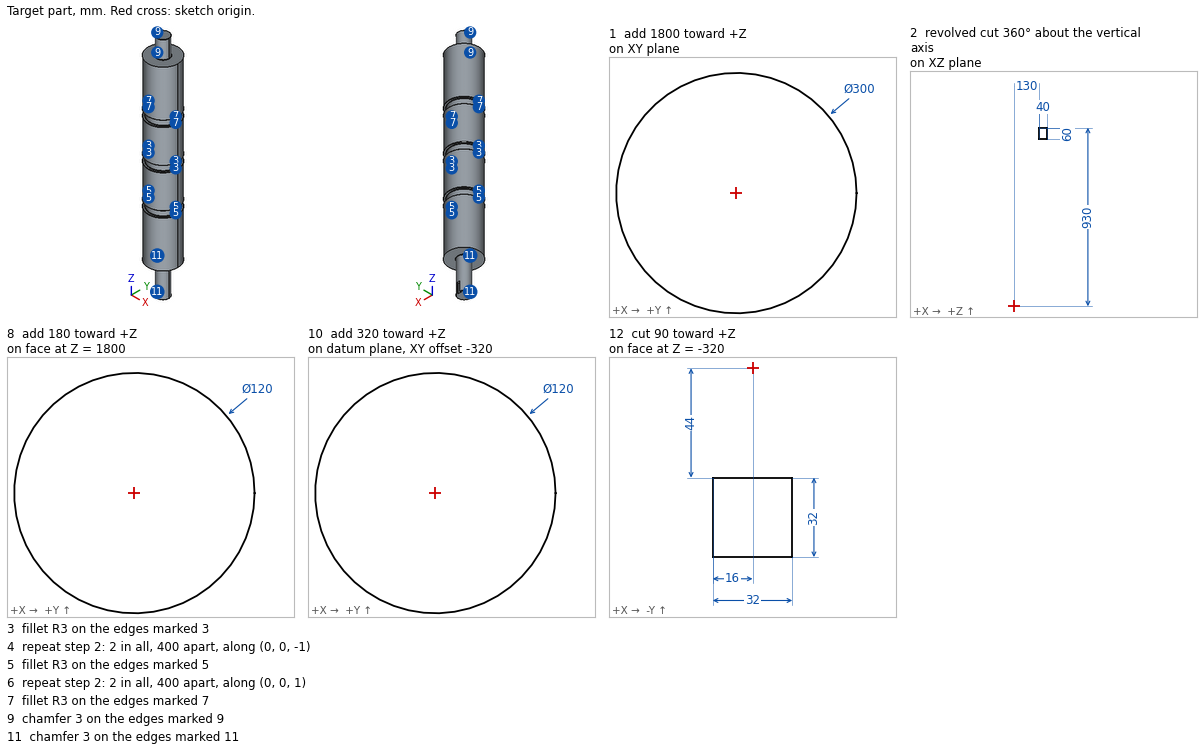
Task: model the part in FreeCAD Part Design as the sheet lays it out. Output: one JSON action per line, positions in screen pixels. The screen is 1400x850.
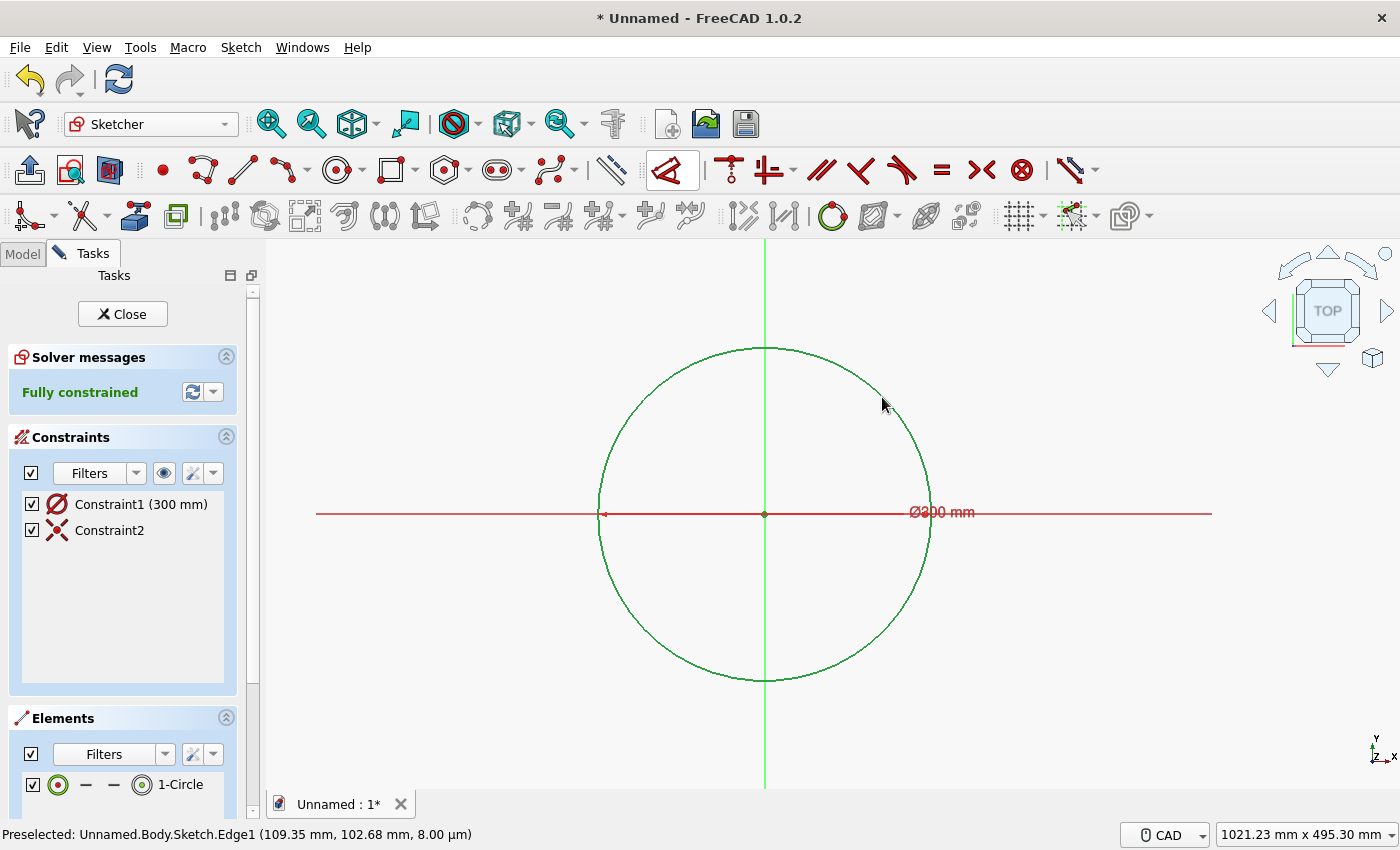
{"action": "left_click", "coordinate": [123, 314]}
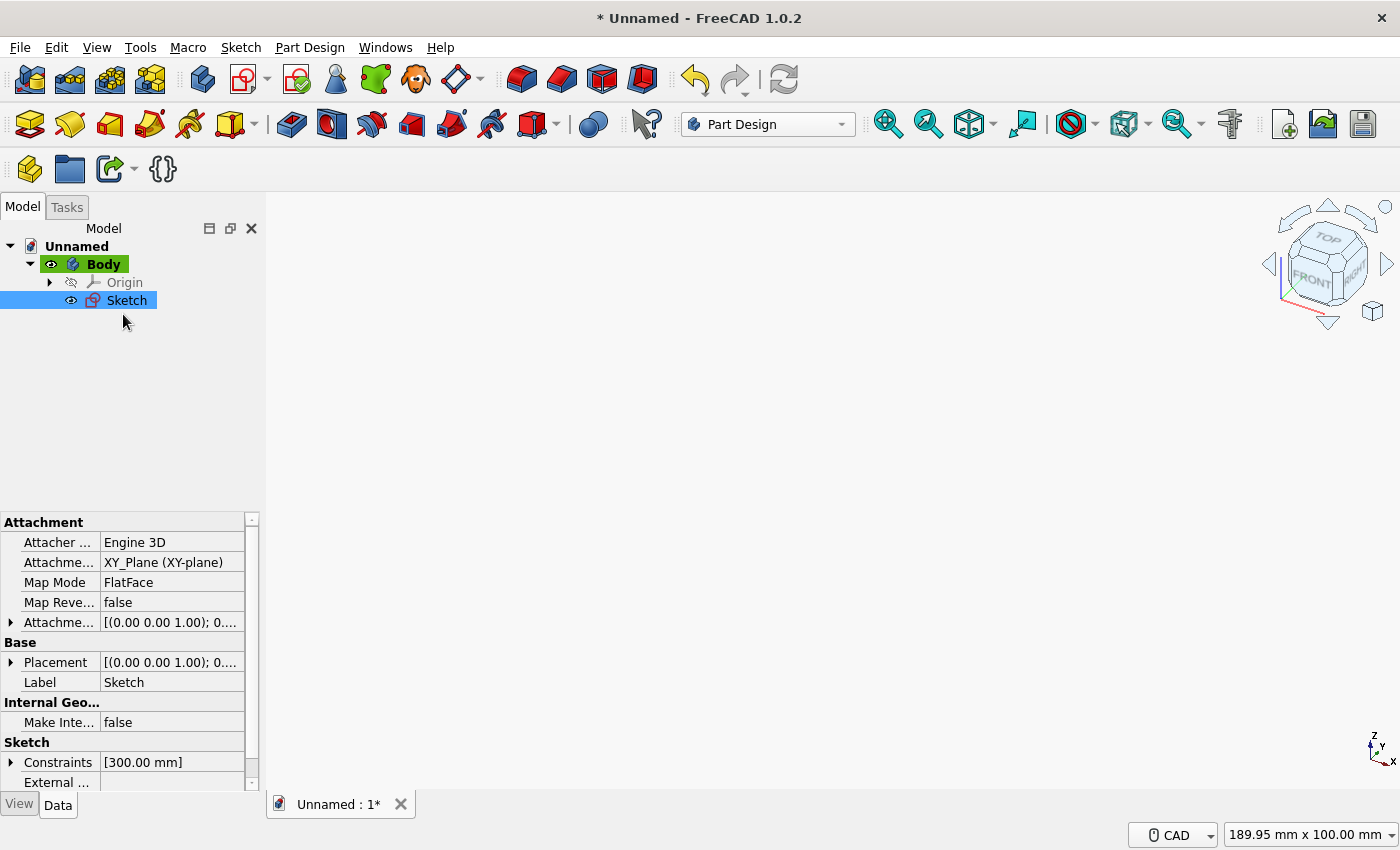
{"action": "left_click", "coordinate": [30, 124]}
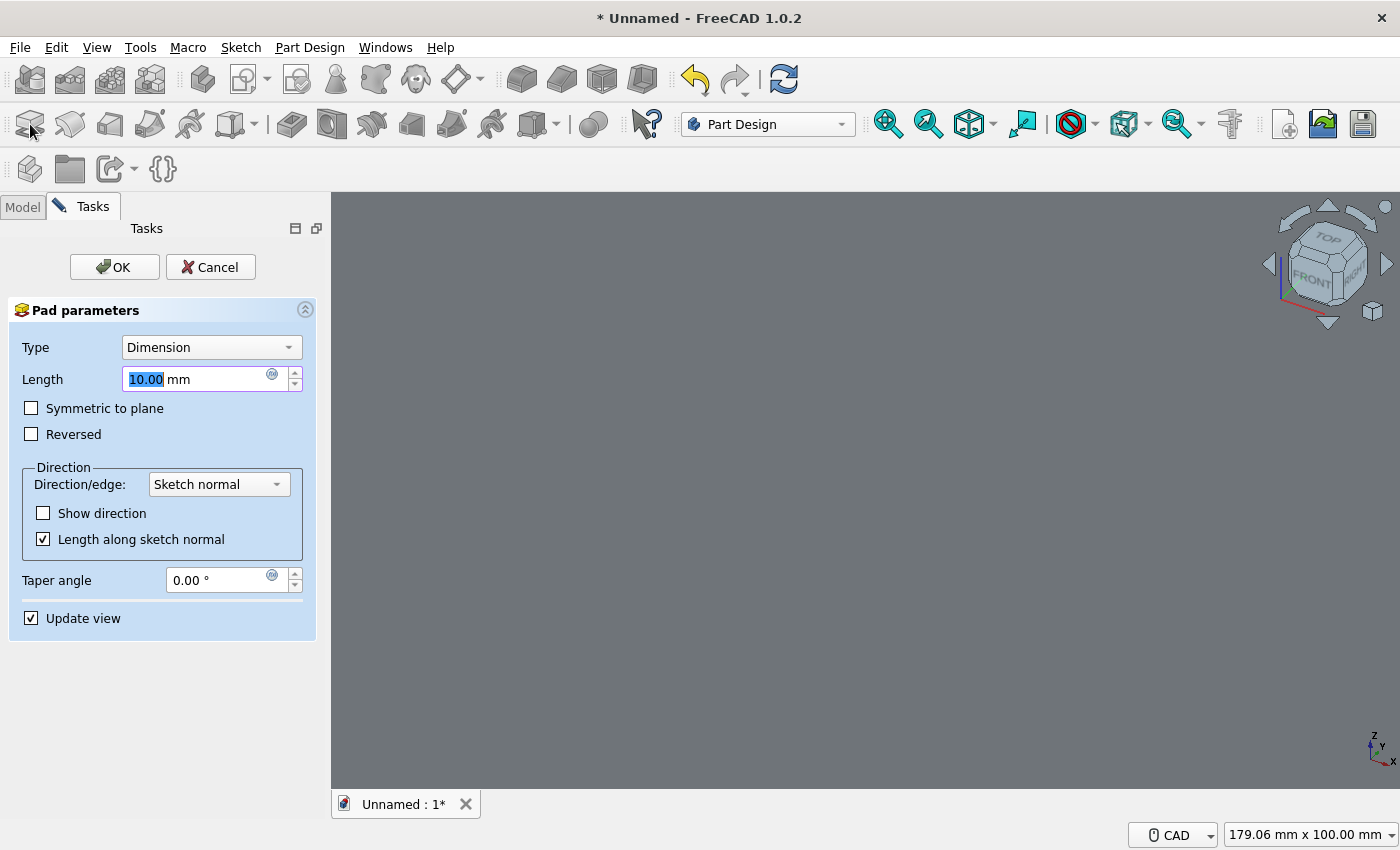
{"action": "type", "text": "1800"}
{"action": "key", "text": "Tab"}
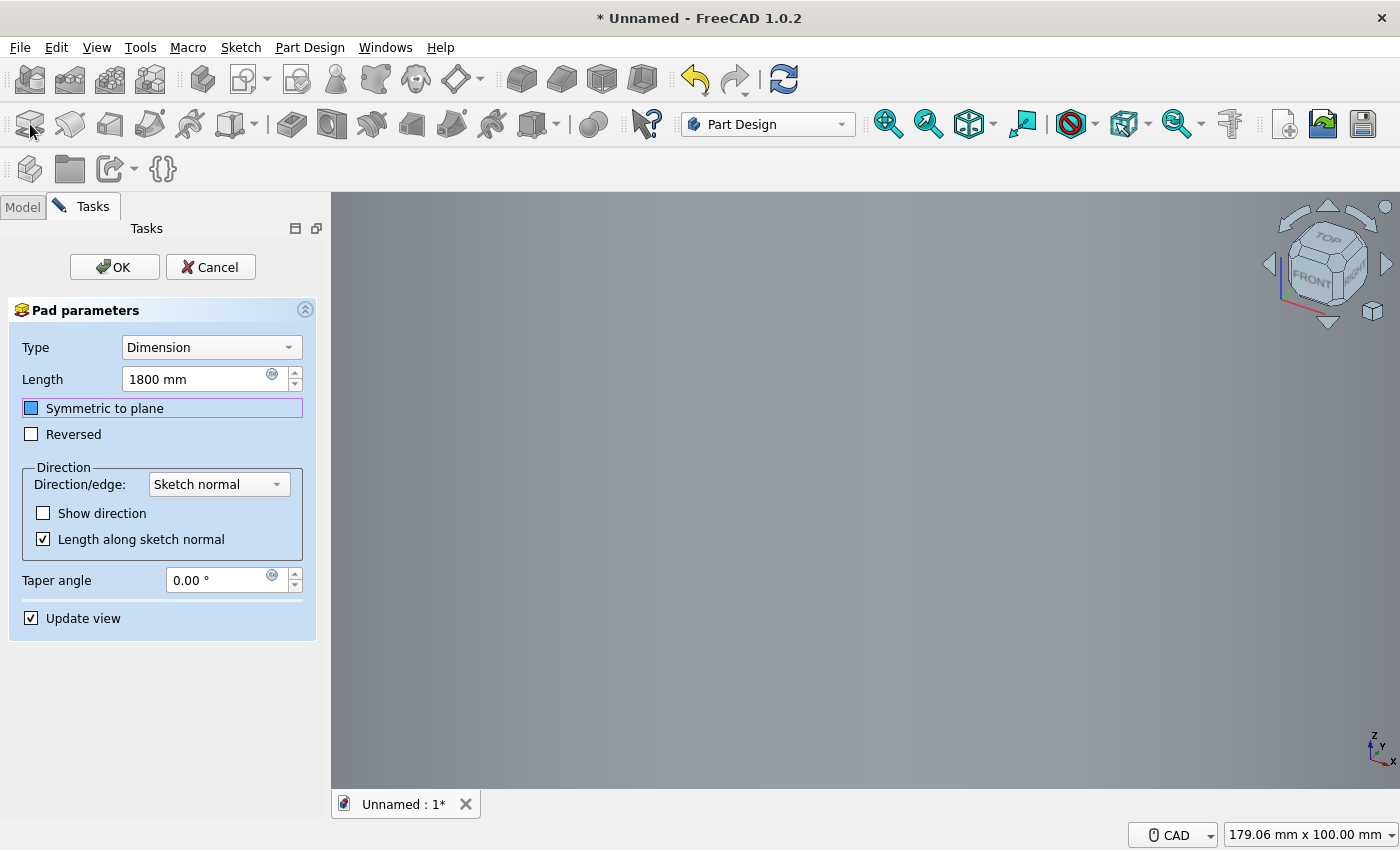
{"action": "left_click", "coordinate": [115, 267]}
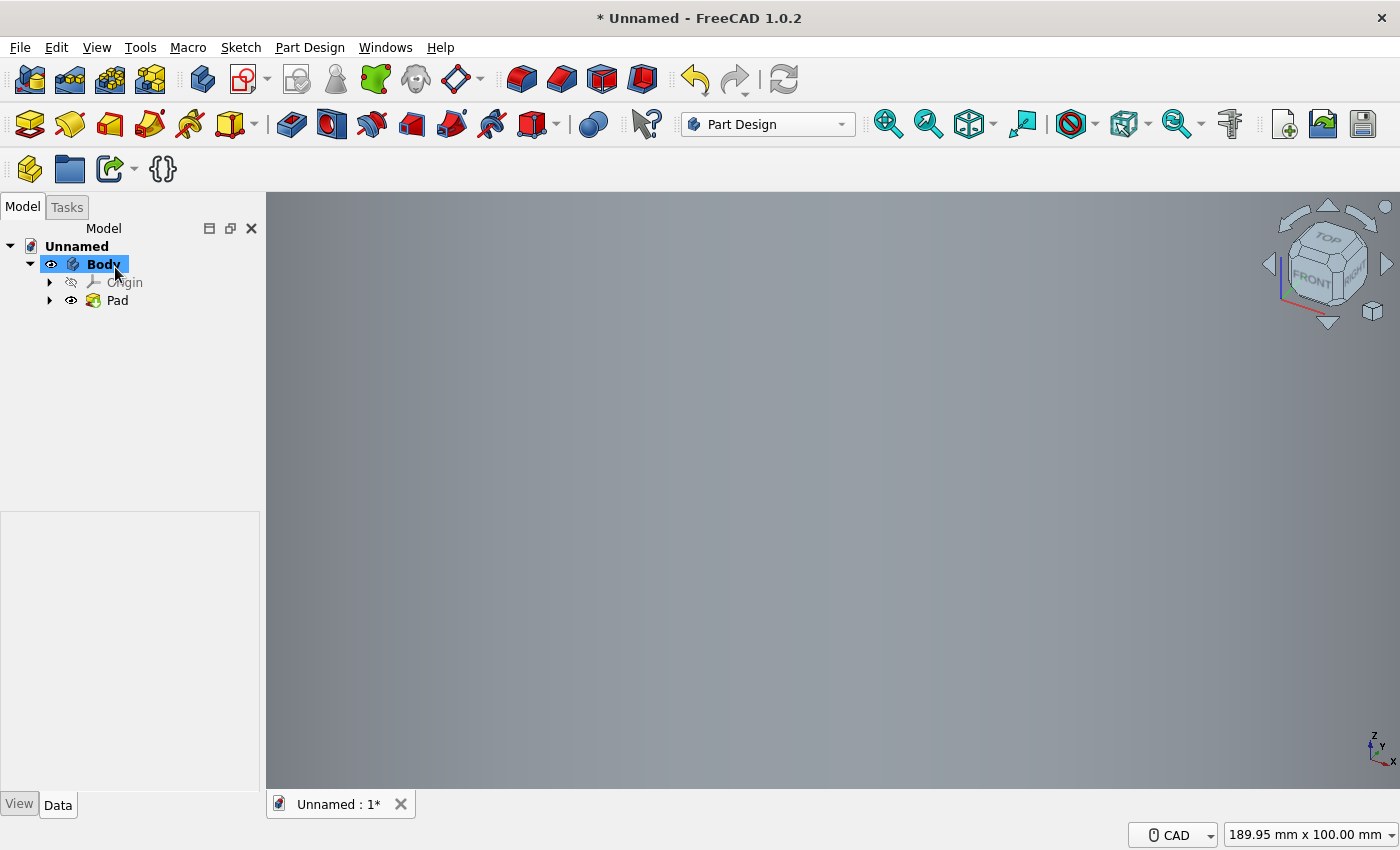
{"action": "left_click", "coordinate": [890, 124]}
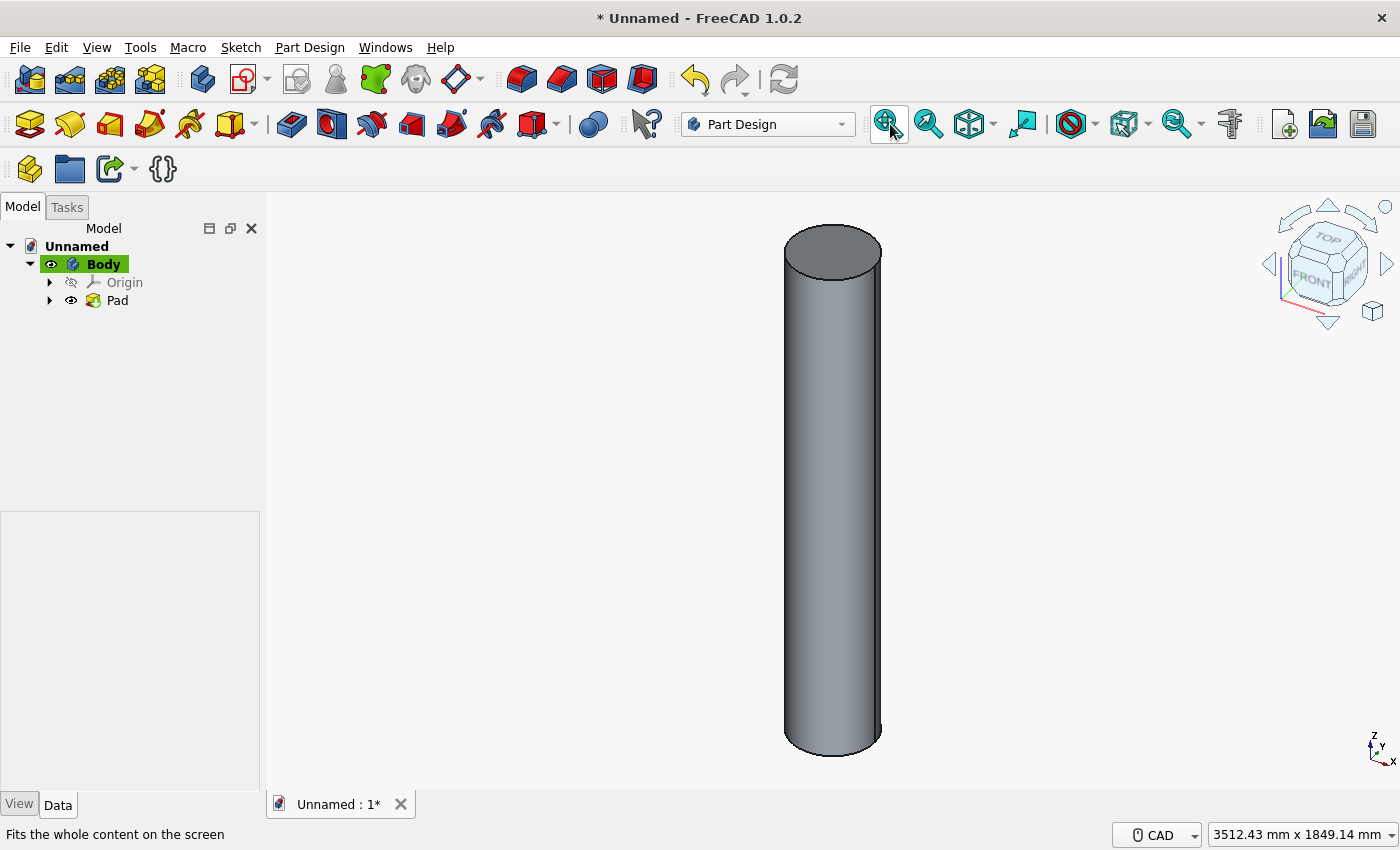
{"action": "left_click", "coordinate": [244, 80]}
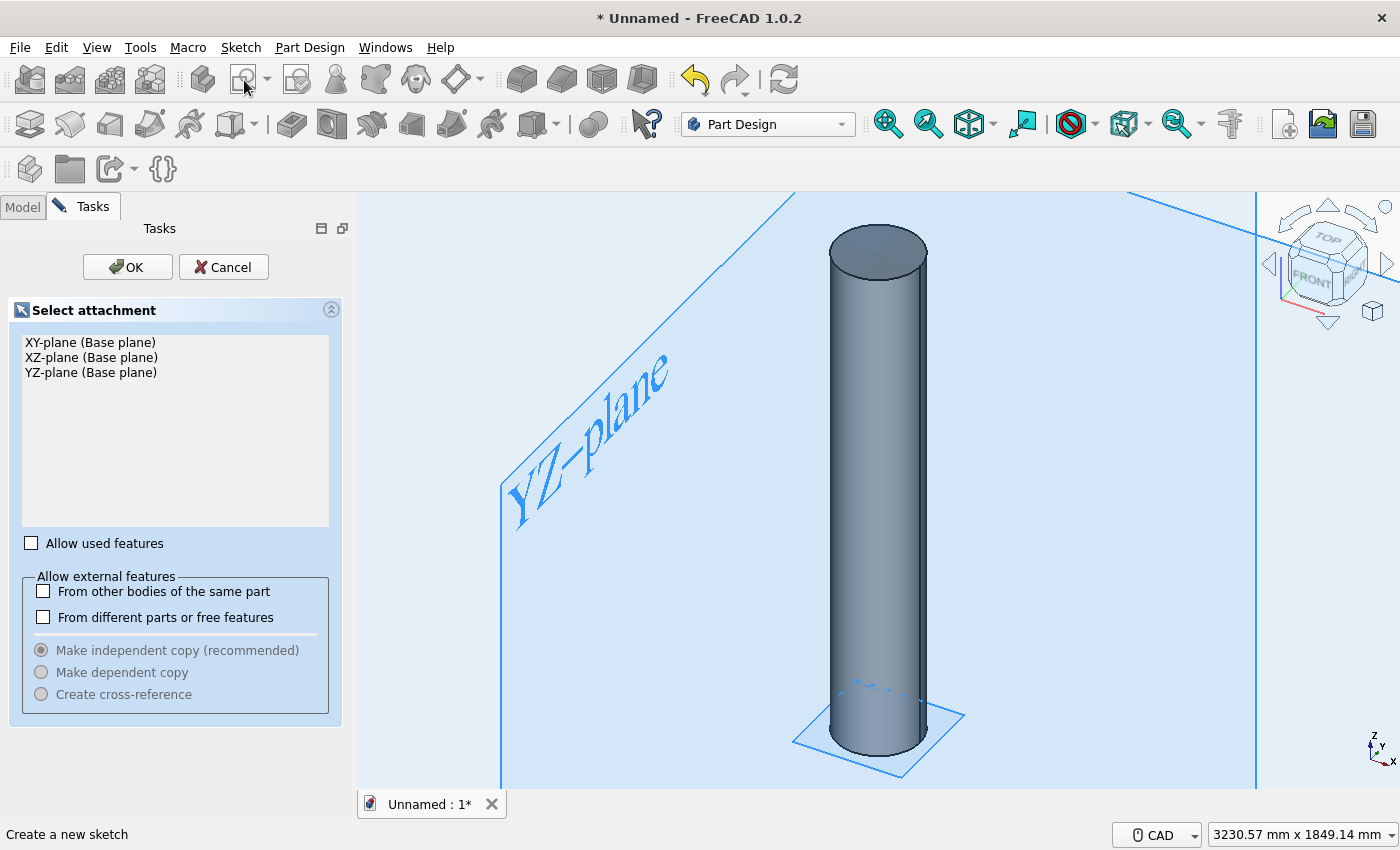
{"action": "left_click", "coordinate": [82, 358]}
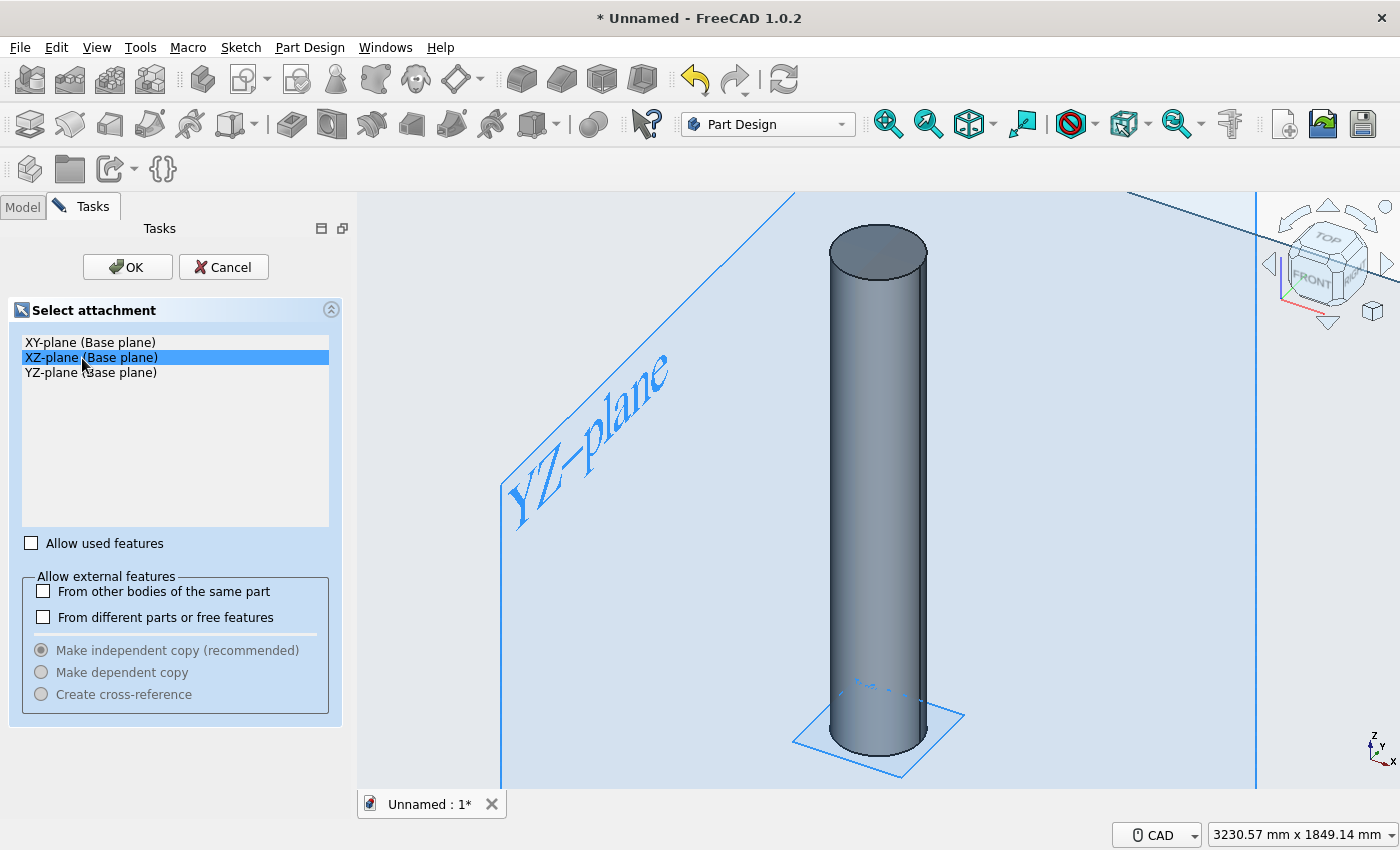
{"action": "left_click", "coordinate": [128, 267]}